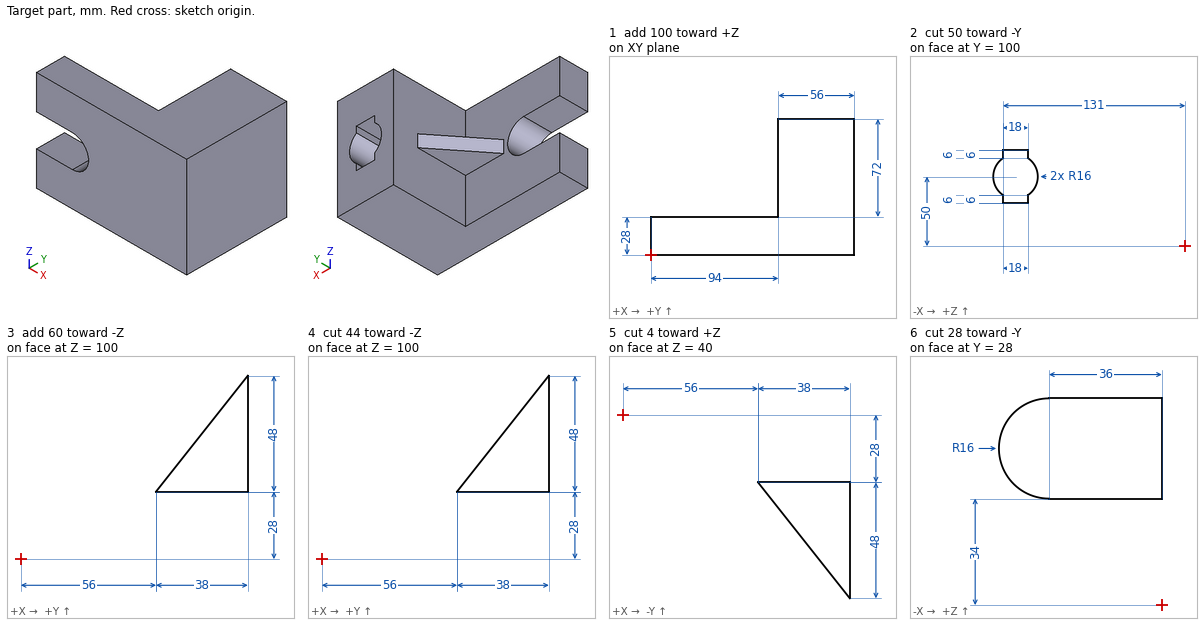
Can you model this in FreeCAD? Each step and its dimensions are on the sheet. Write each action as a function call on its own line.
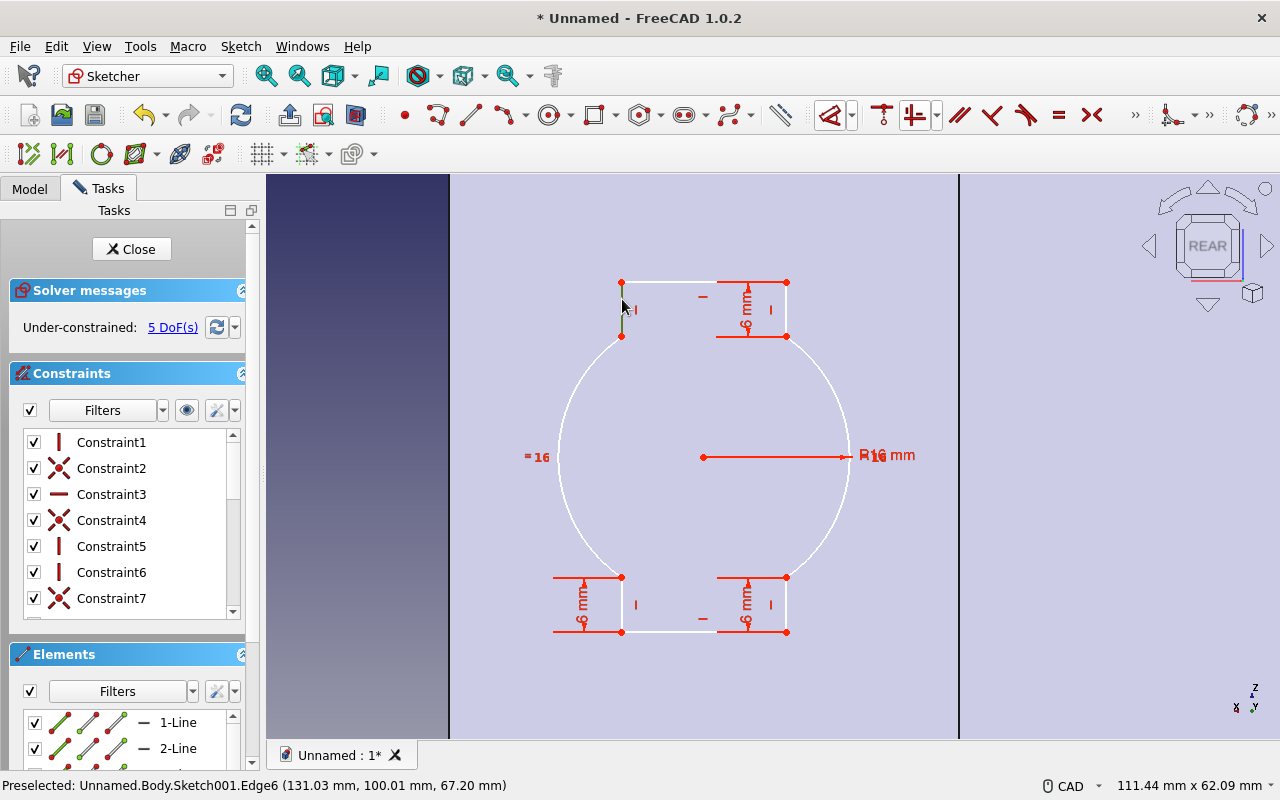
click(852, 116)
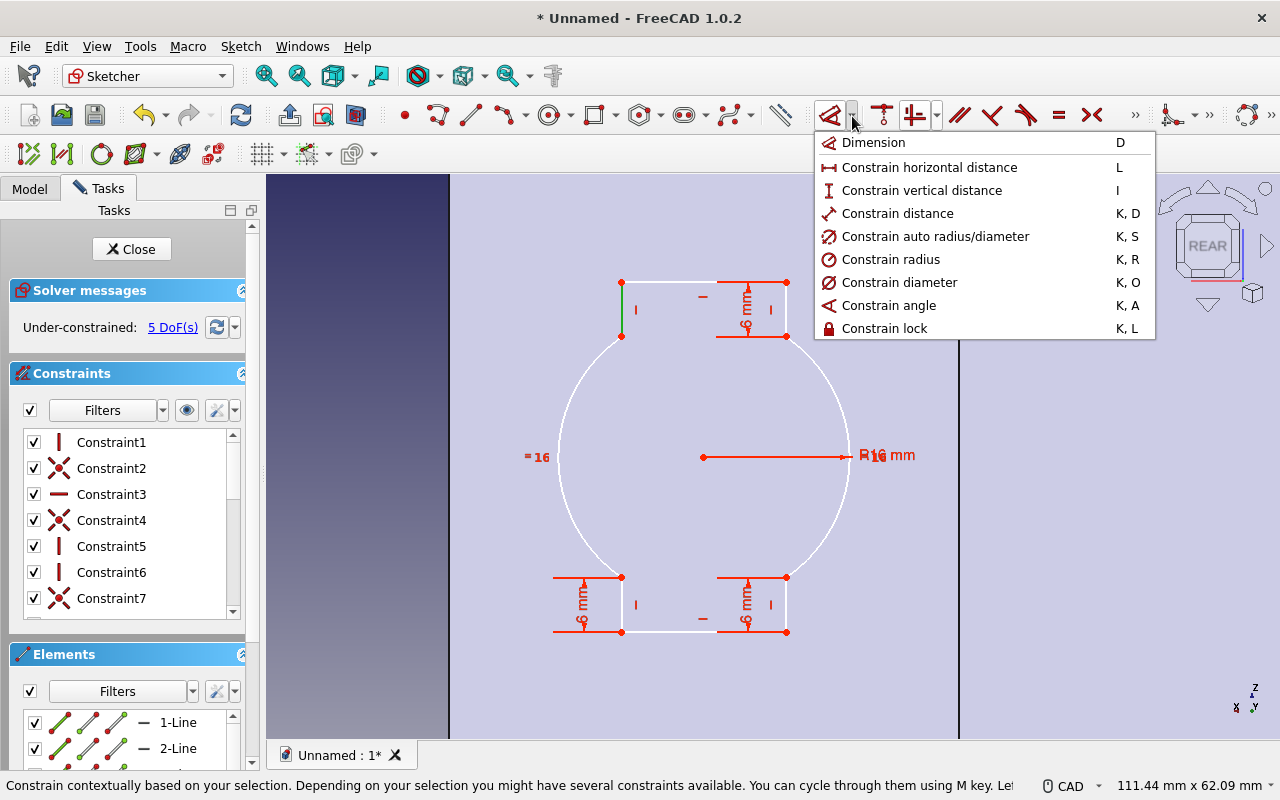
click(985, 190)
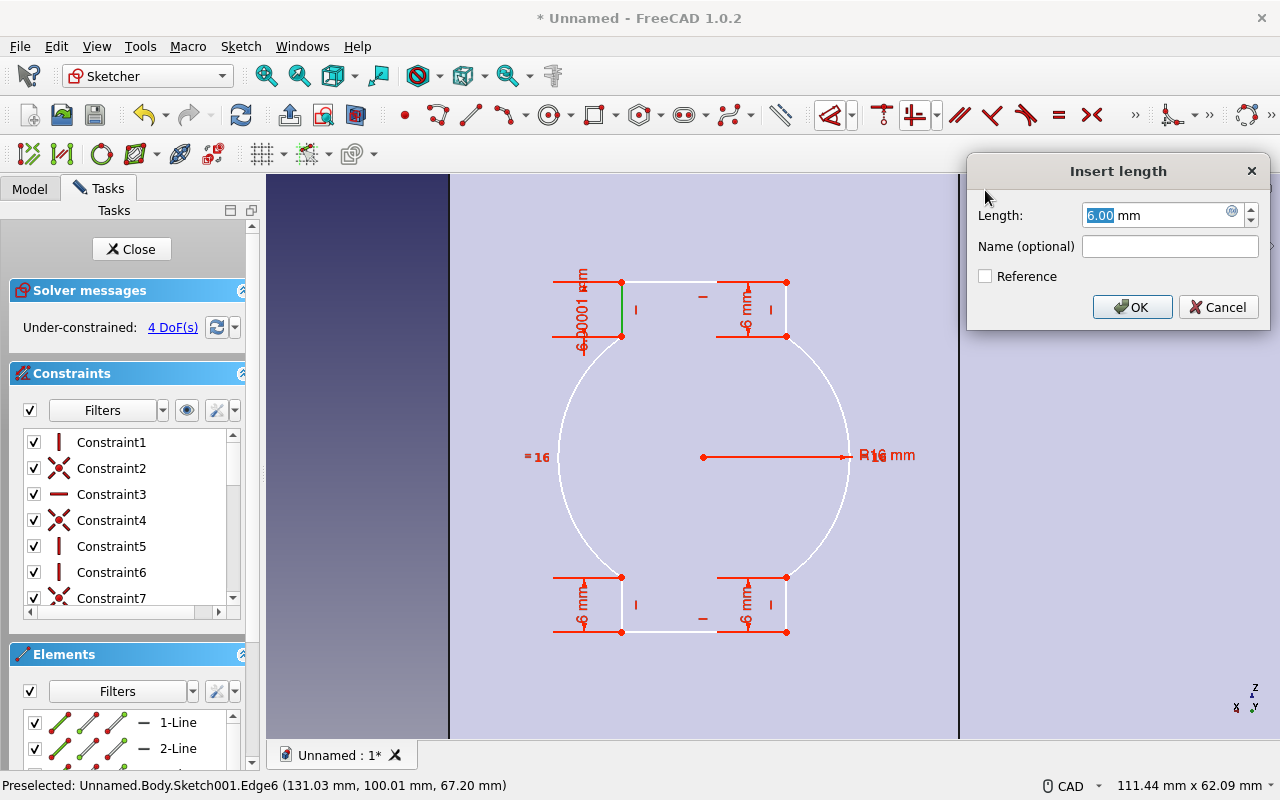
text(6)
key(Return)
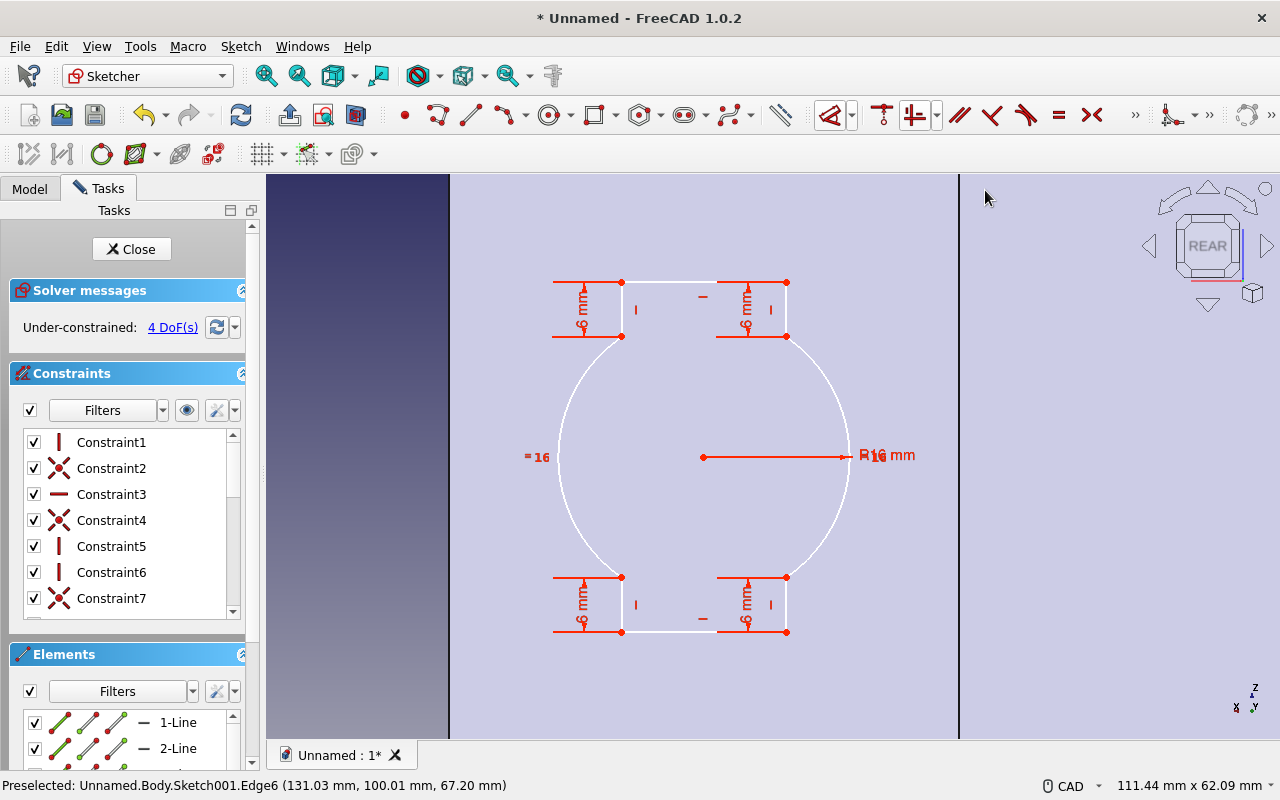
click(671, 632)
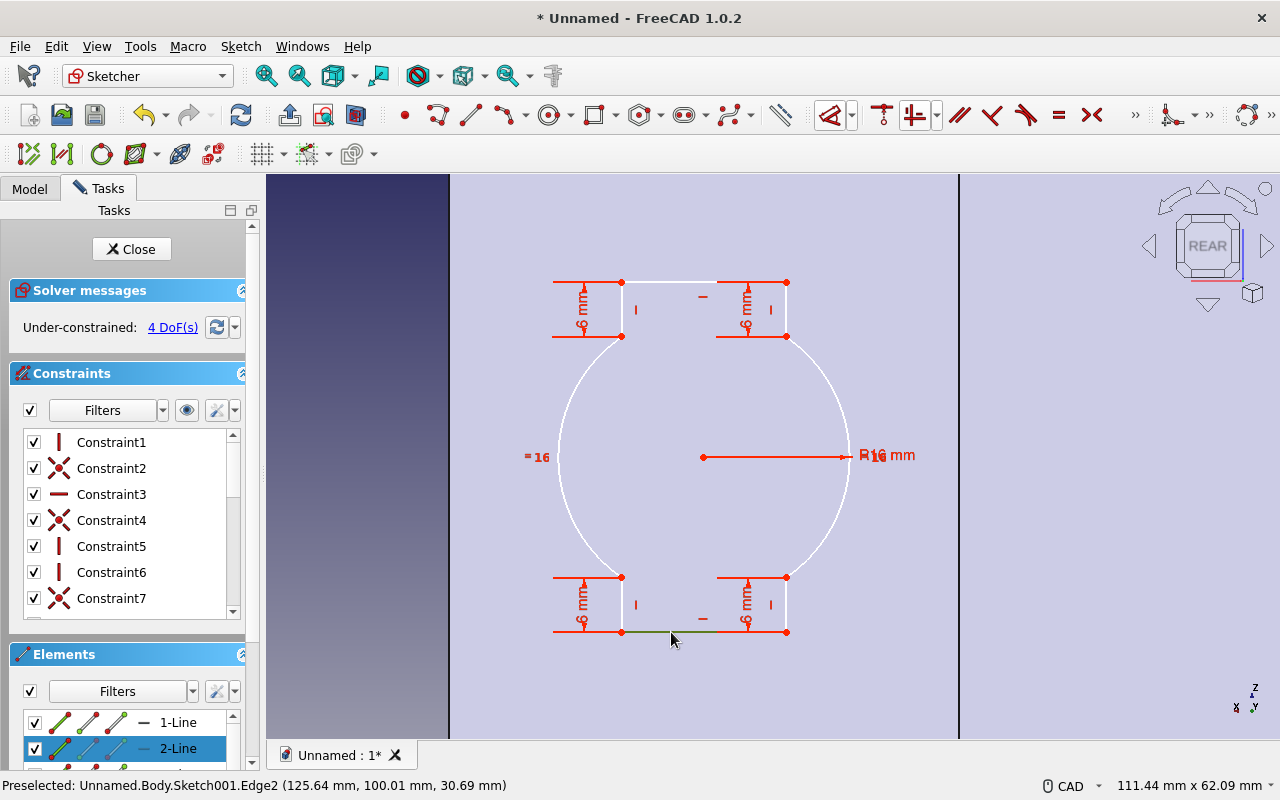
click(852, 116)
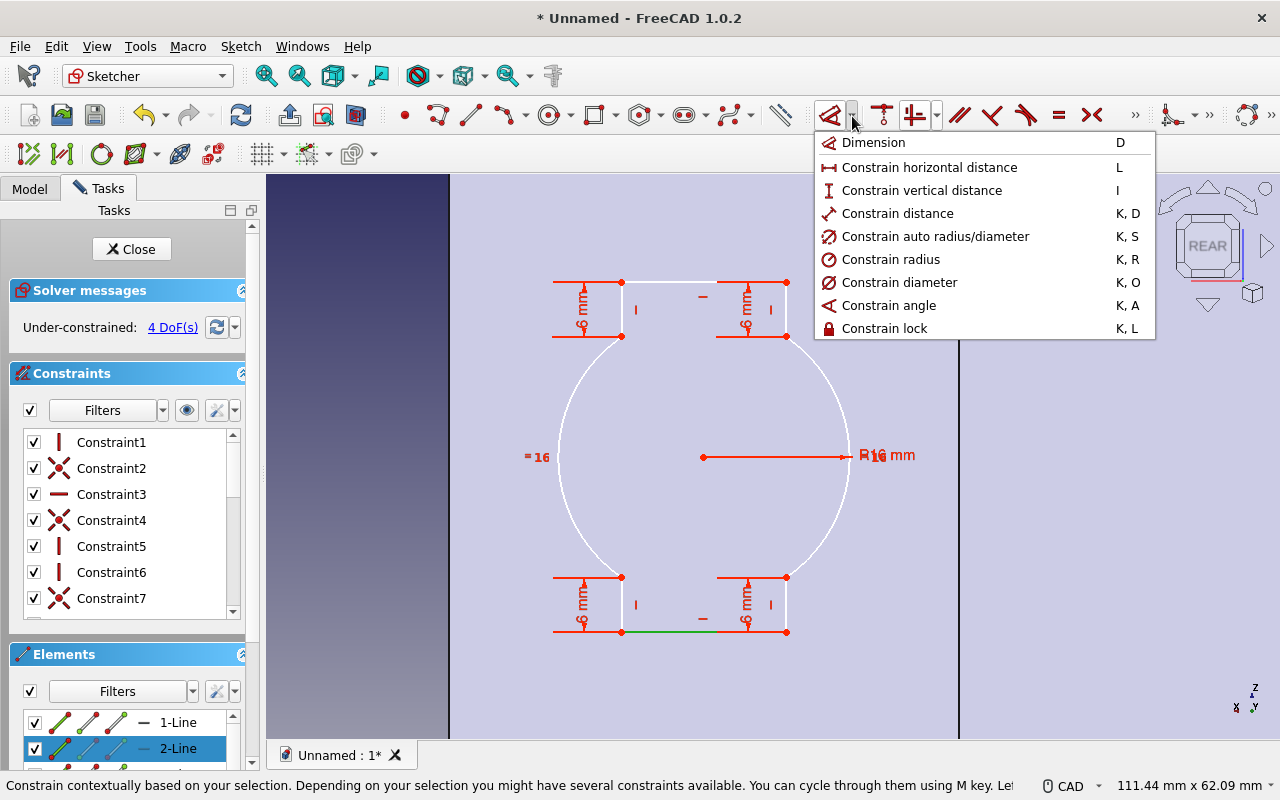
click(985, 168)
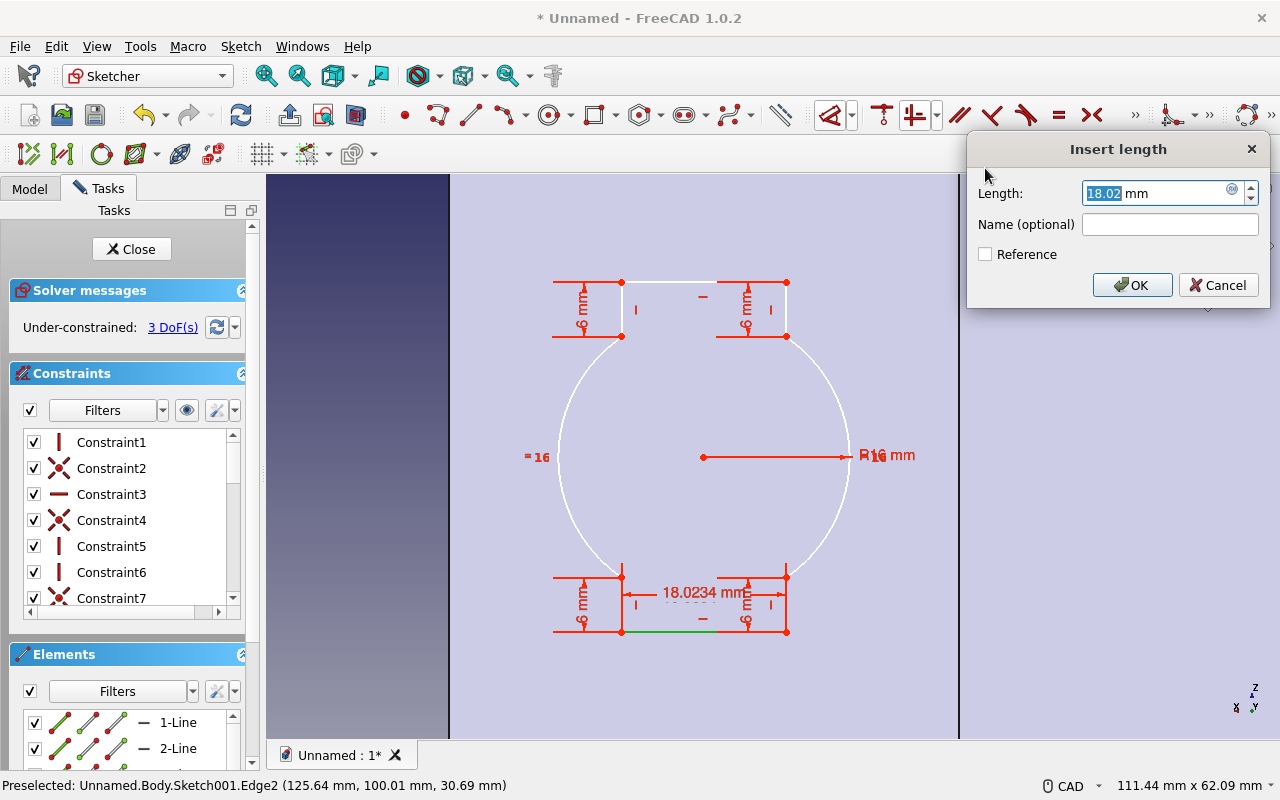
text(18)
key(Return)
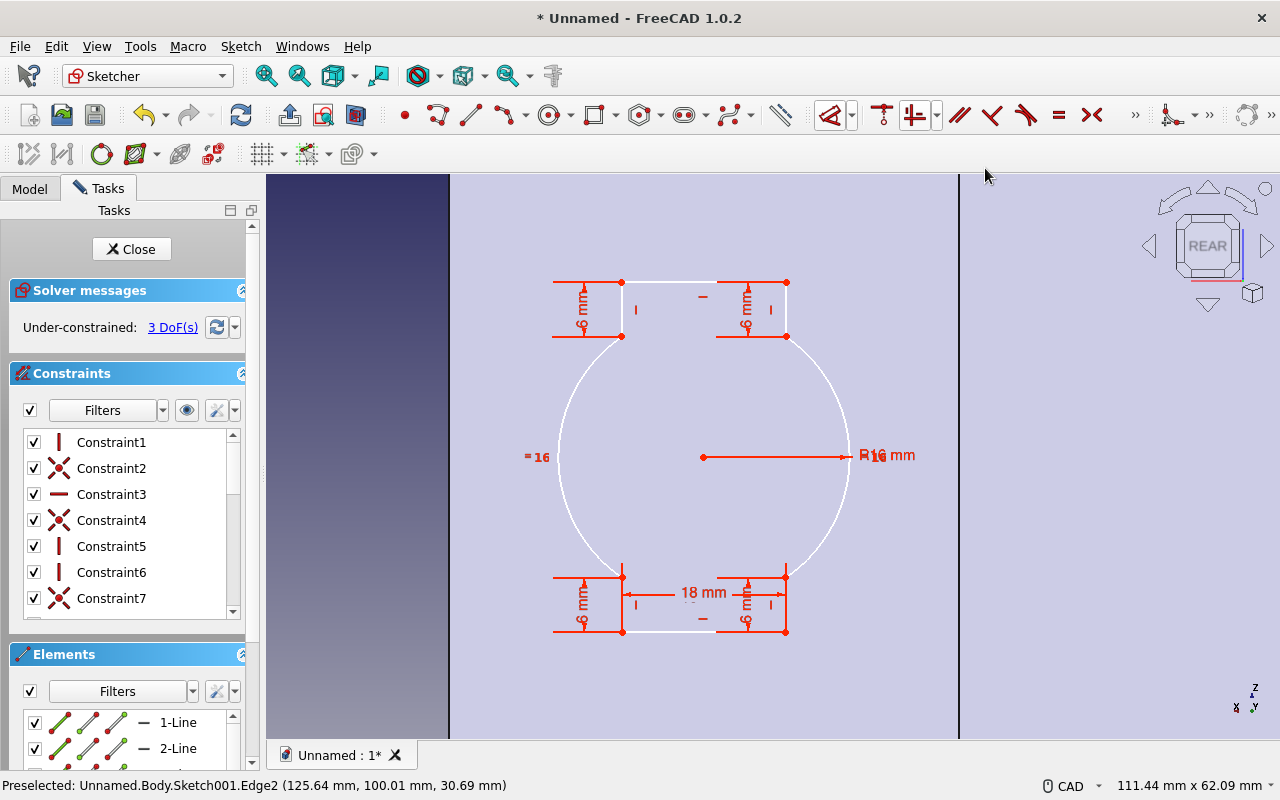
click(737, 282)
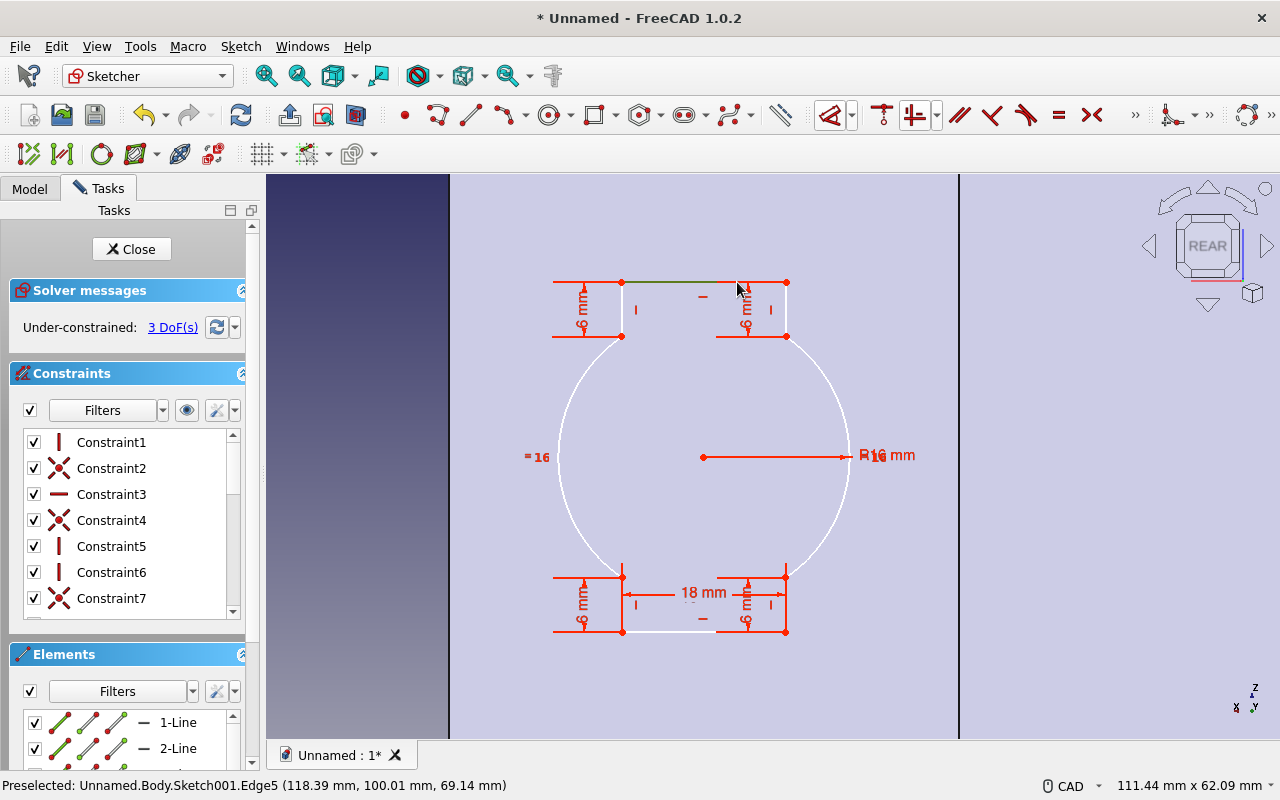
key(l)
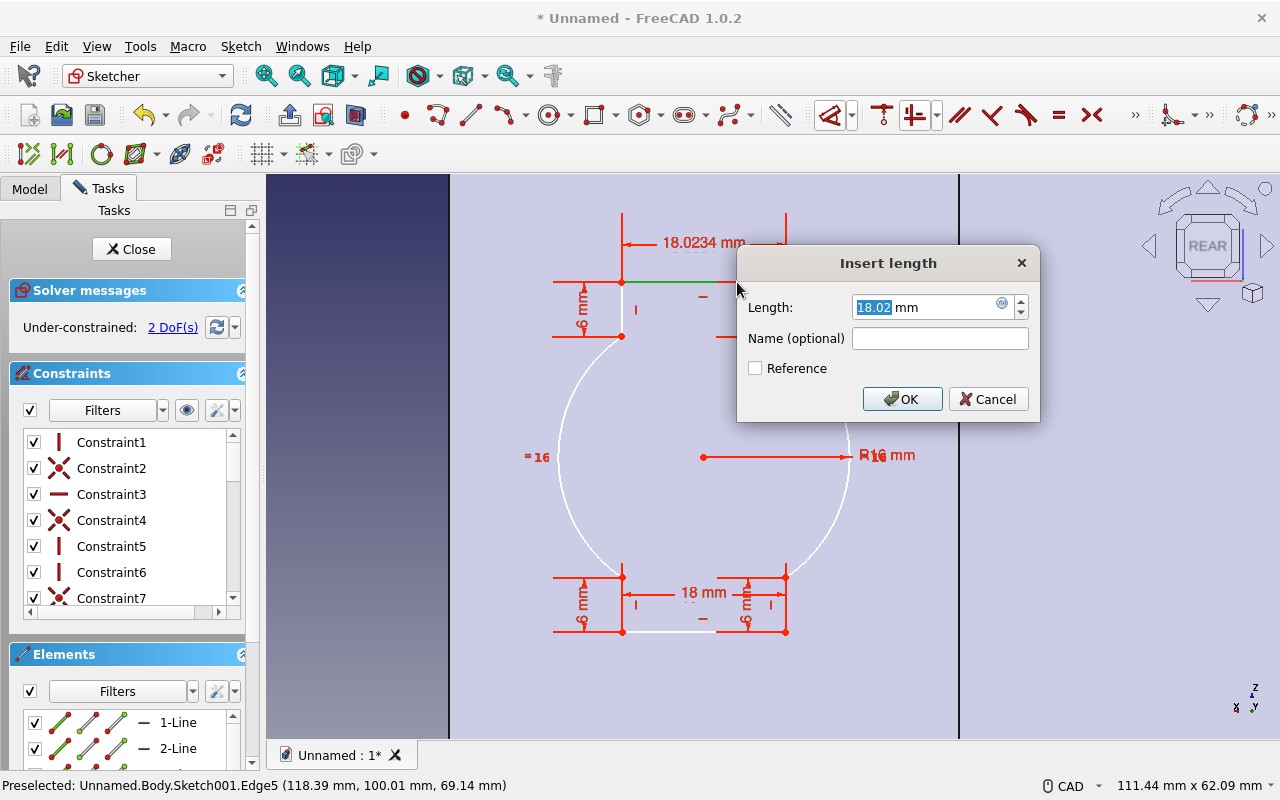
text(18)
key(Return)